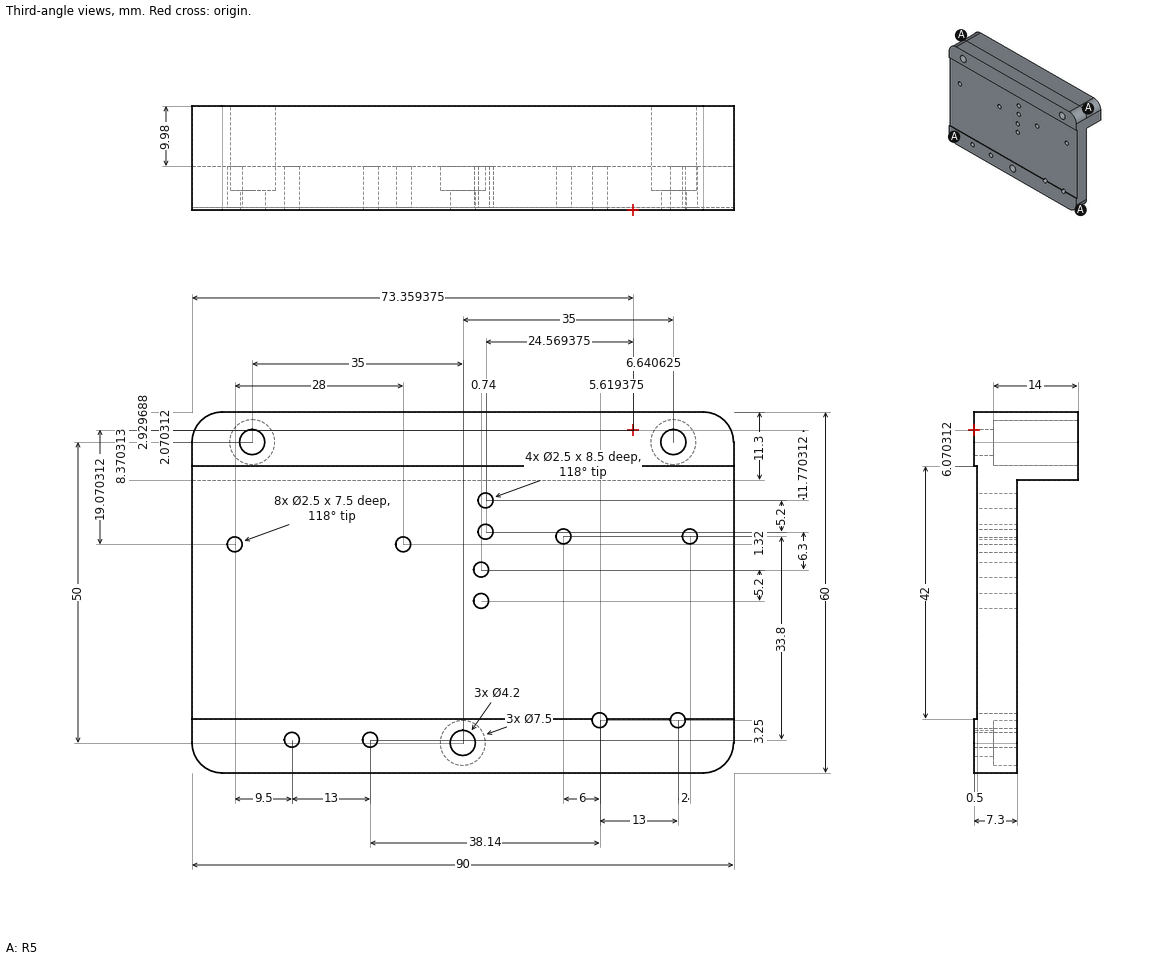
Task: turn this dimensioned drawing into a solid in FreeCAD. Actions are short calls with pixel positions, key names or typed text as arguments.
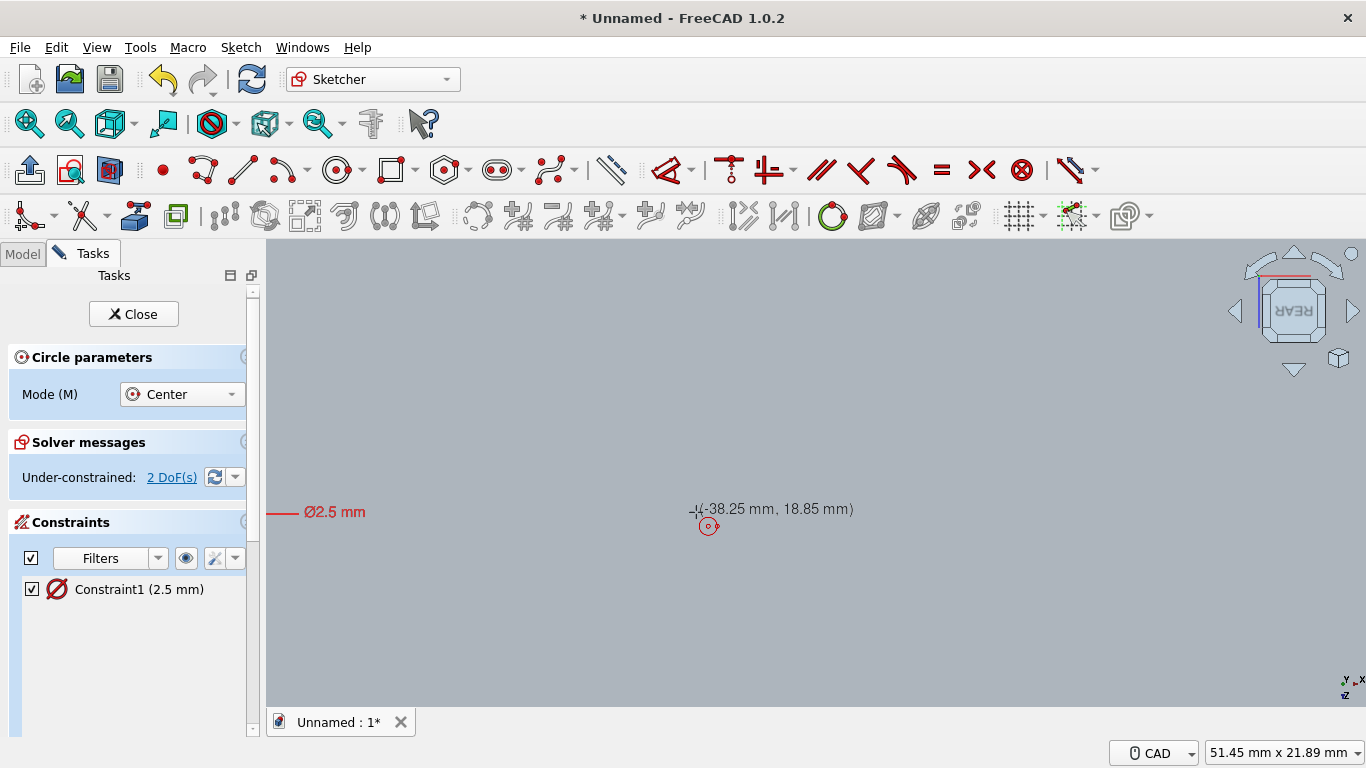
scroll(696, 512, down, 7)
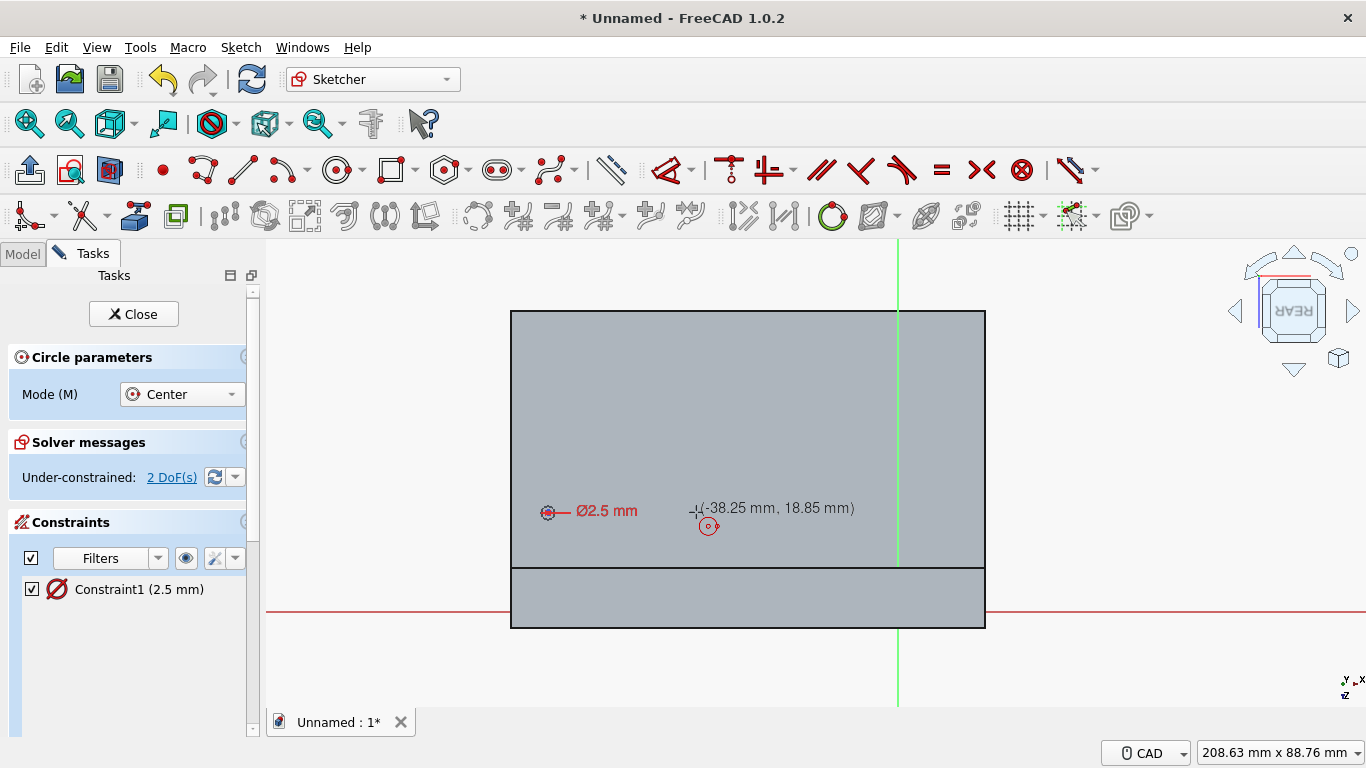
click(696, 512)
move(701, 507)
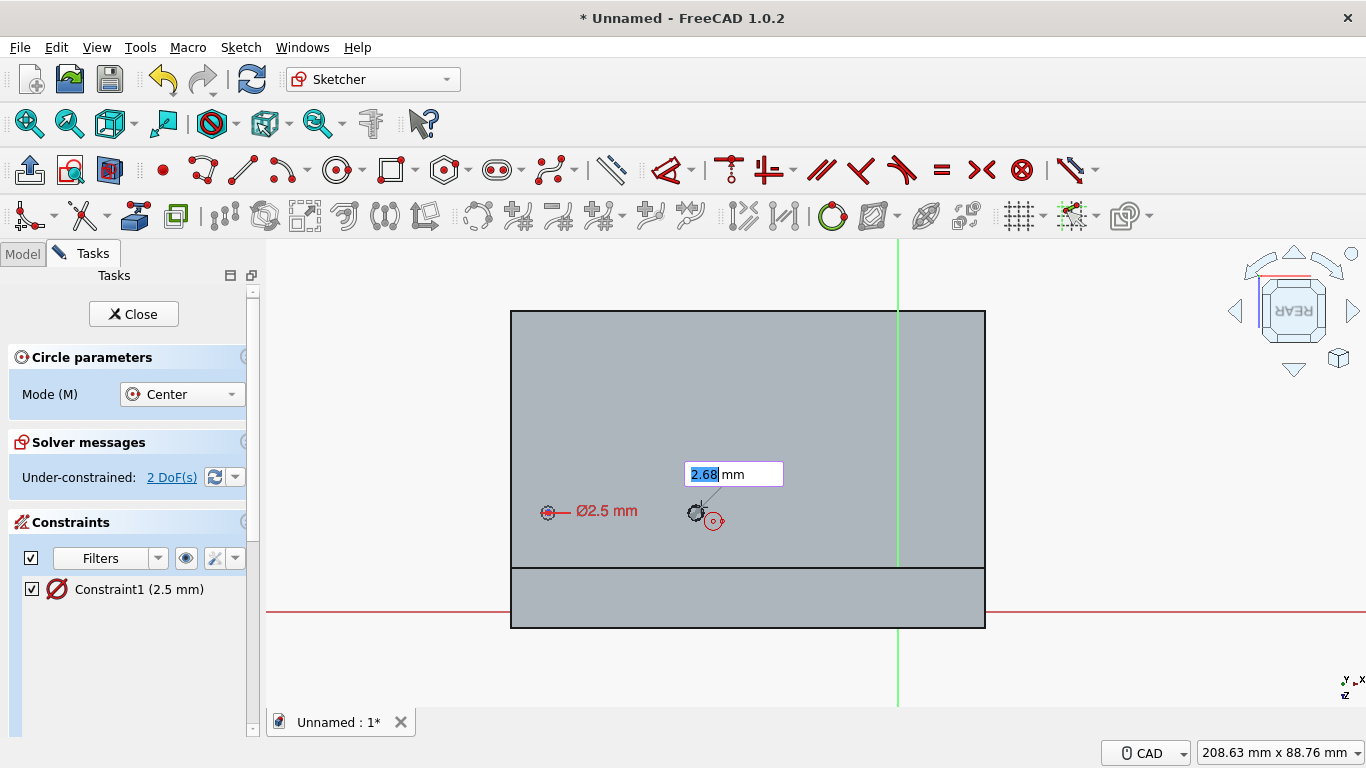
text(2.5)
key(Return)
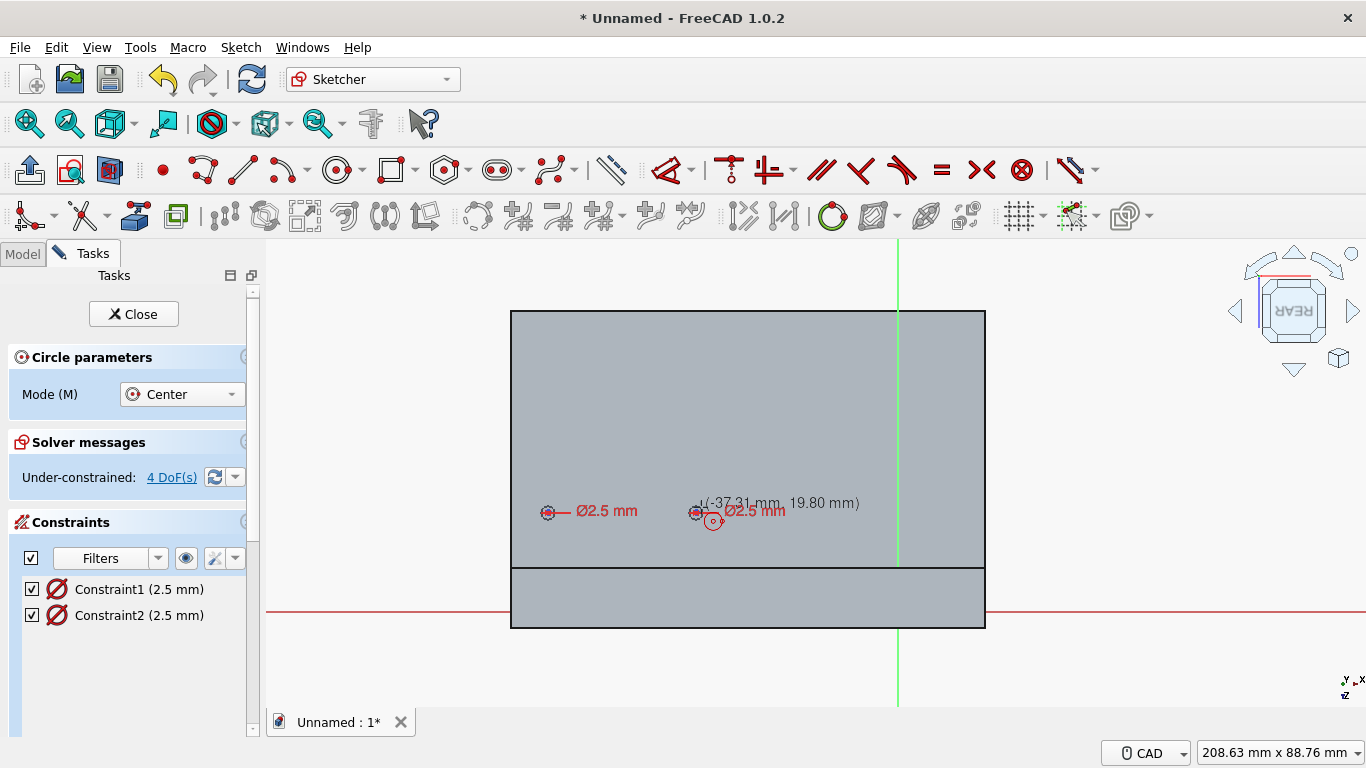
scroll(598, 341, up, 7)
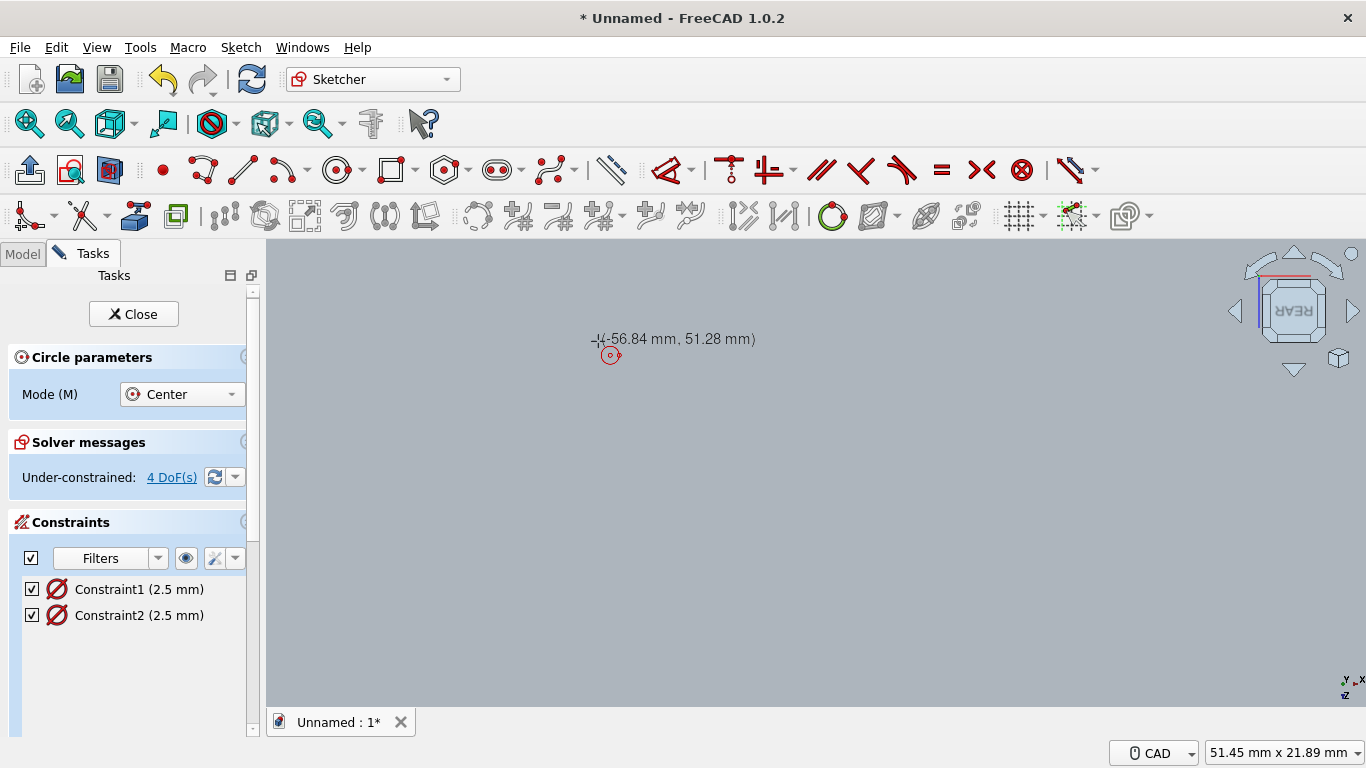
scroll(598, 341, down, 7)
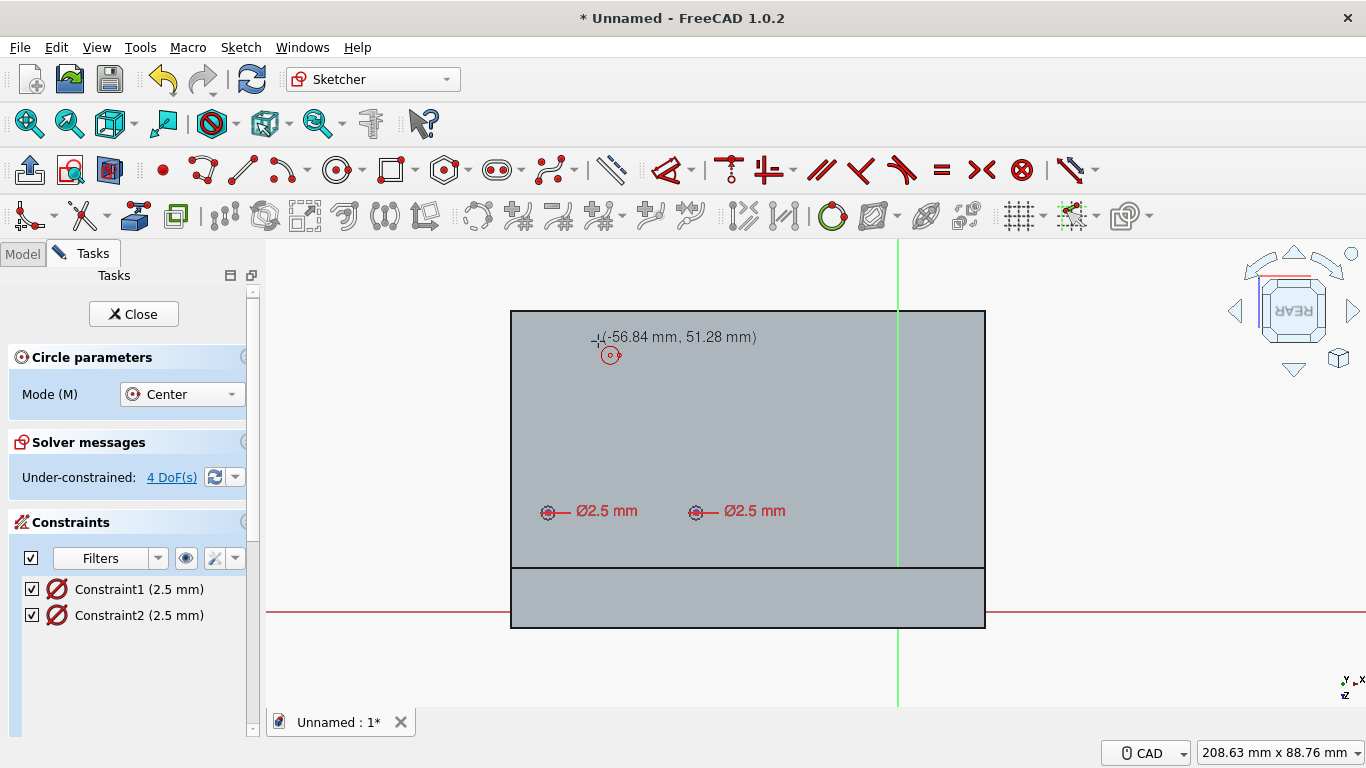
click(598, 341)
move(603, 336)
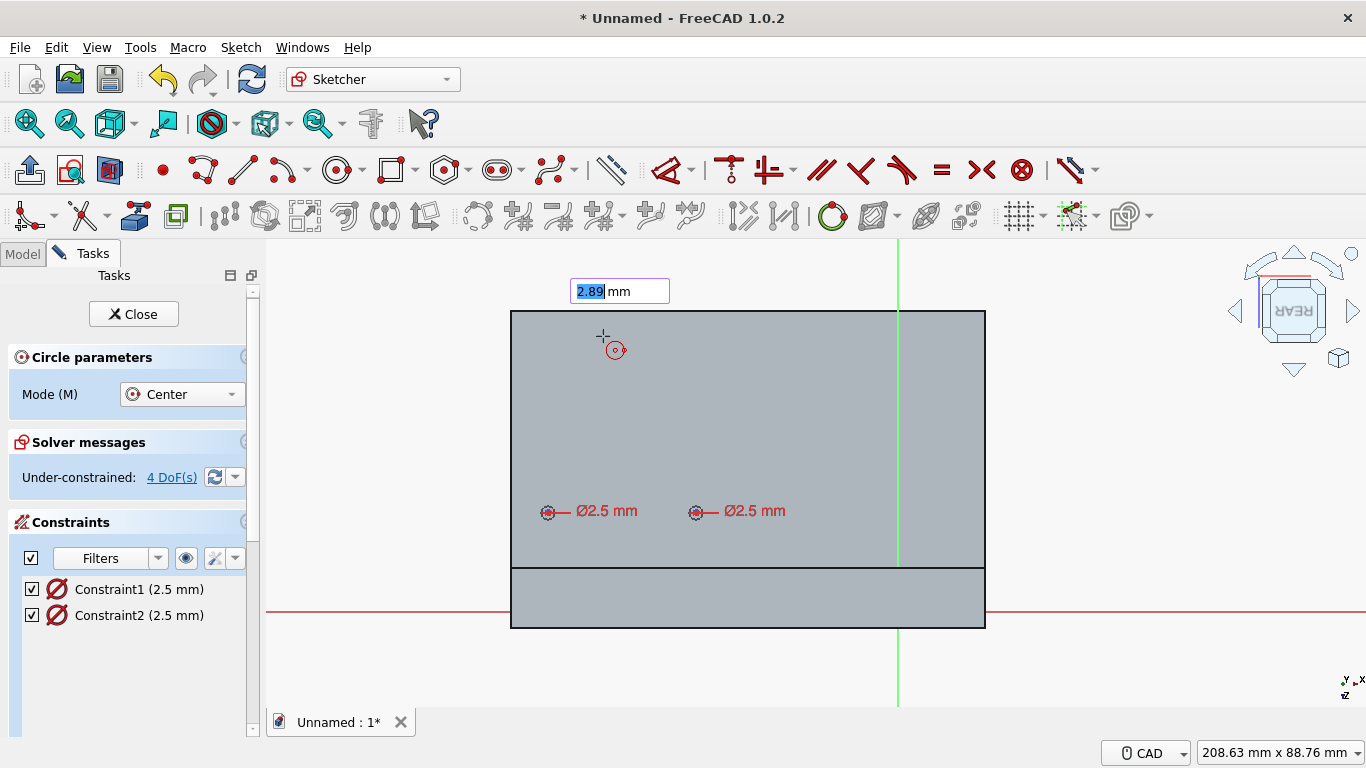
text(2.5)
key(Return)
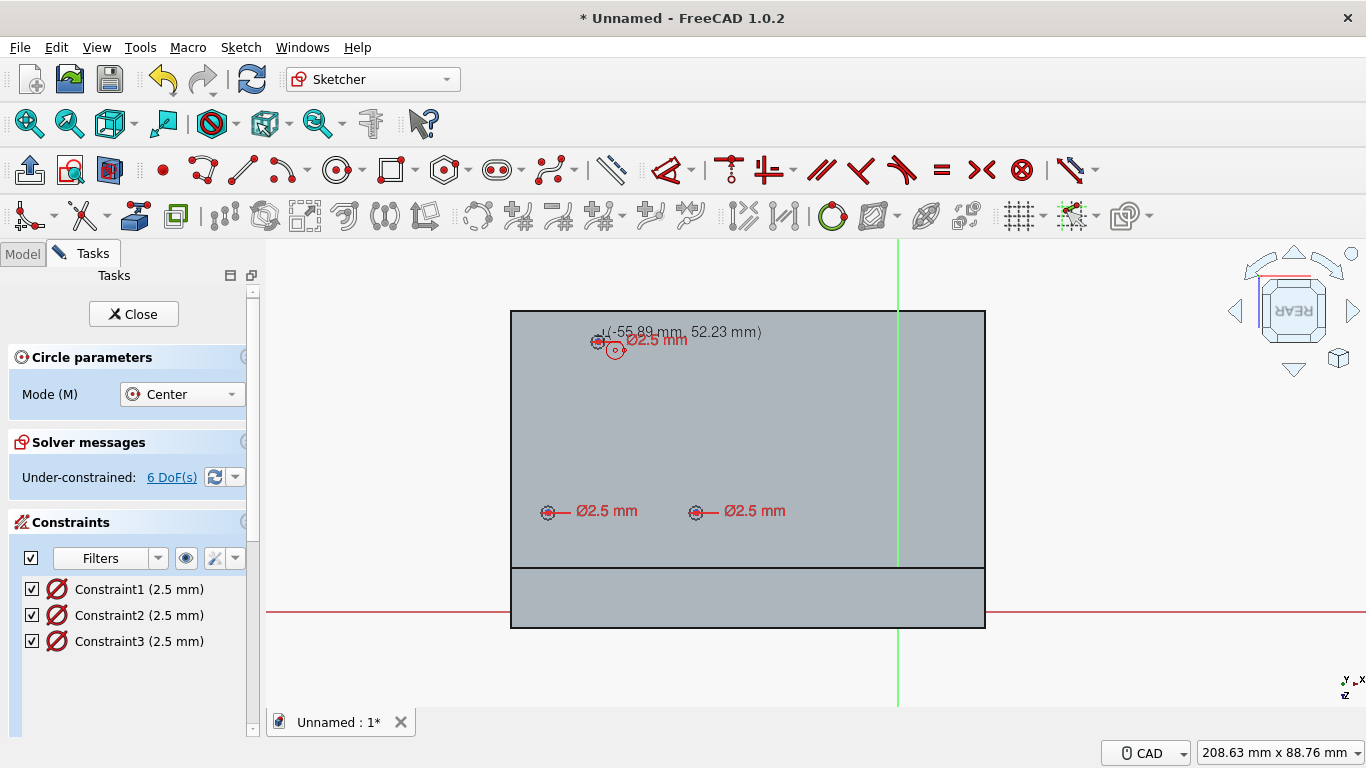
scroll(667, 341, up, 7)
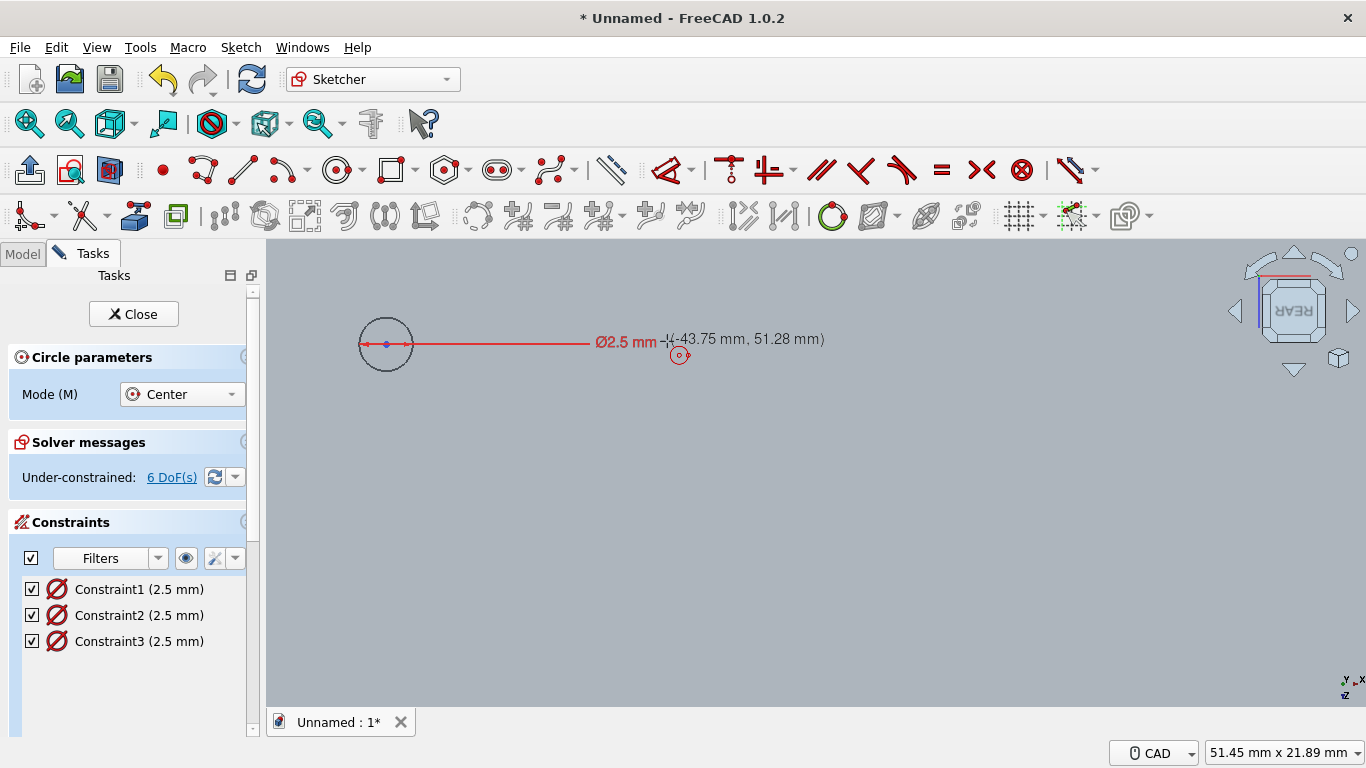
scroll(667, 341, down, 7)